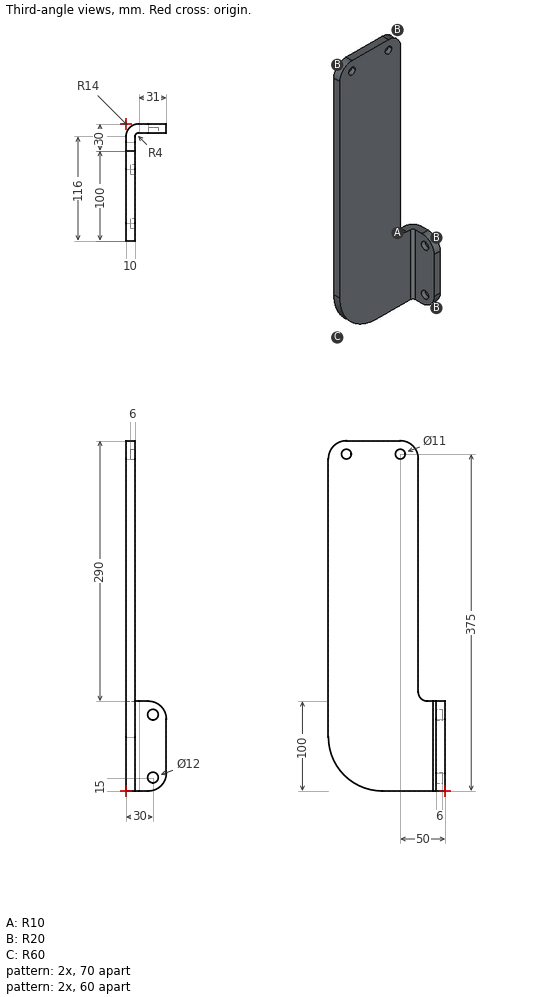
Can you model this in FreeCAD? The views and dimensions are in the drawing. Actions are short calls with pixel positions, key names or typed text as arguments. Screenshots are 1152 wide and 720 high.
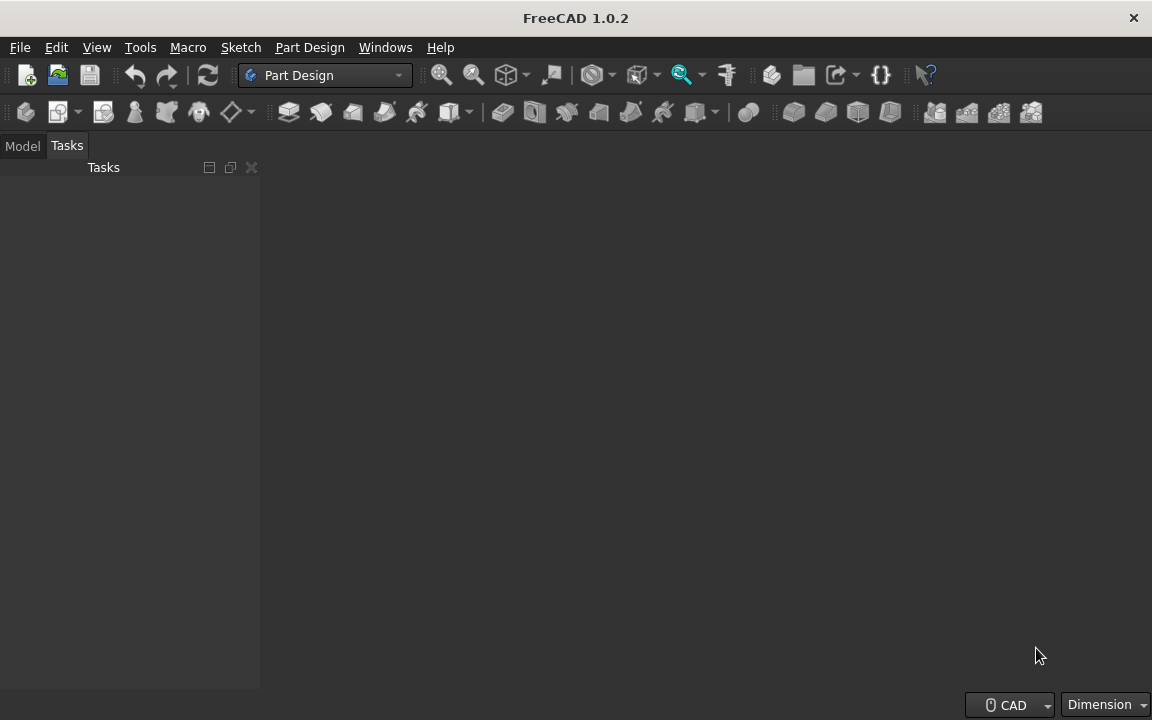
click(26, 76)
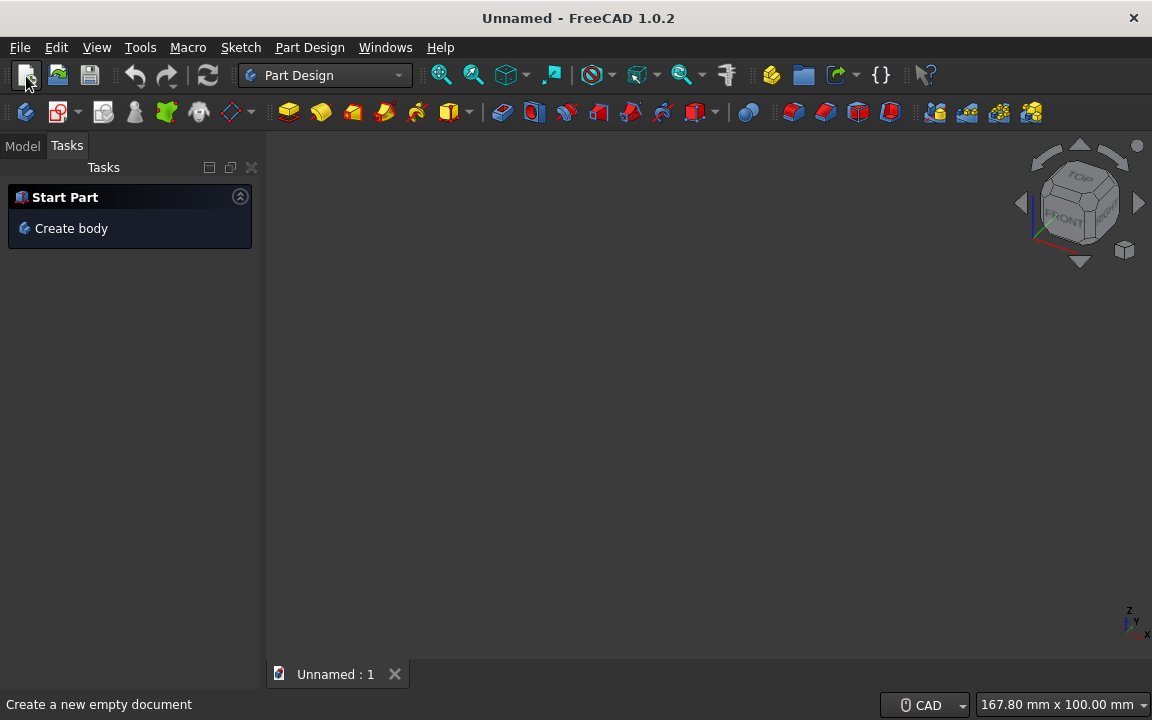
click(58, 112)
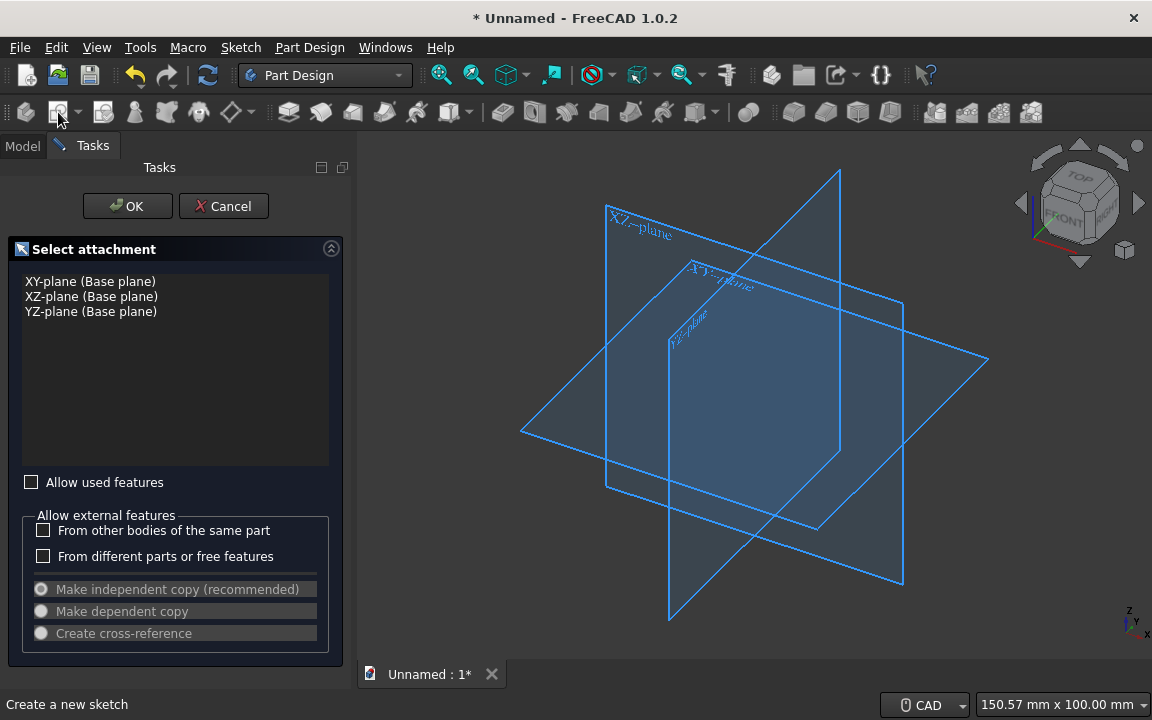
click(82, 282)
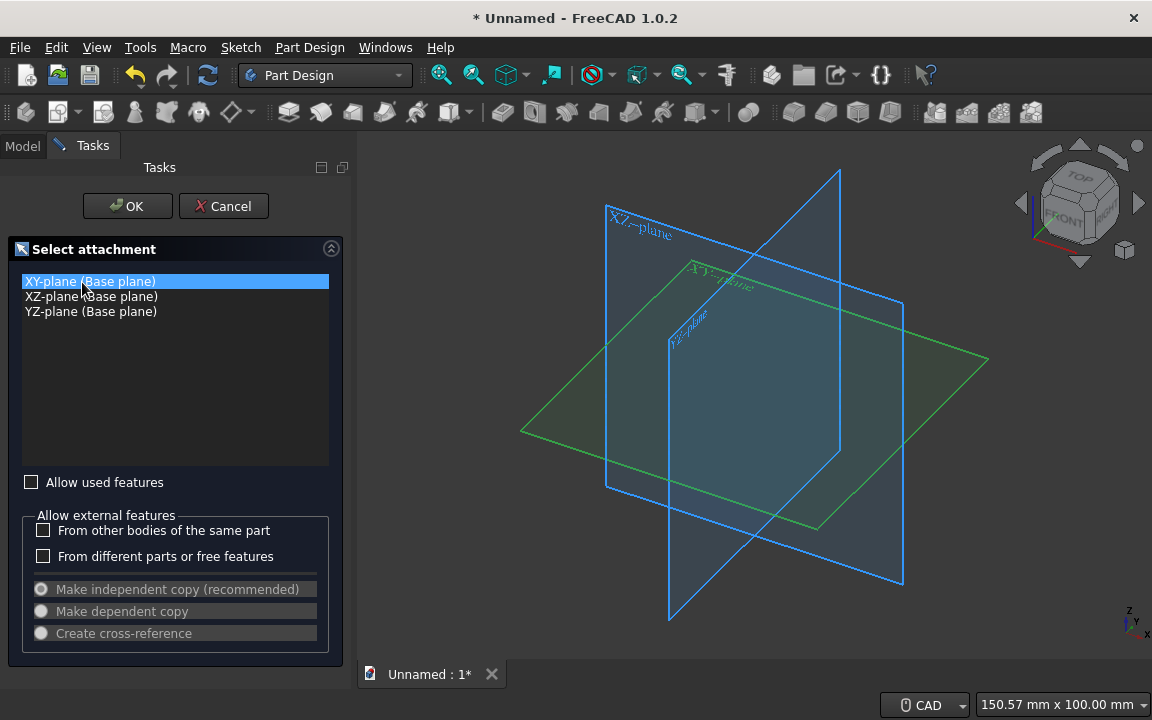
click(128, 206)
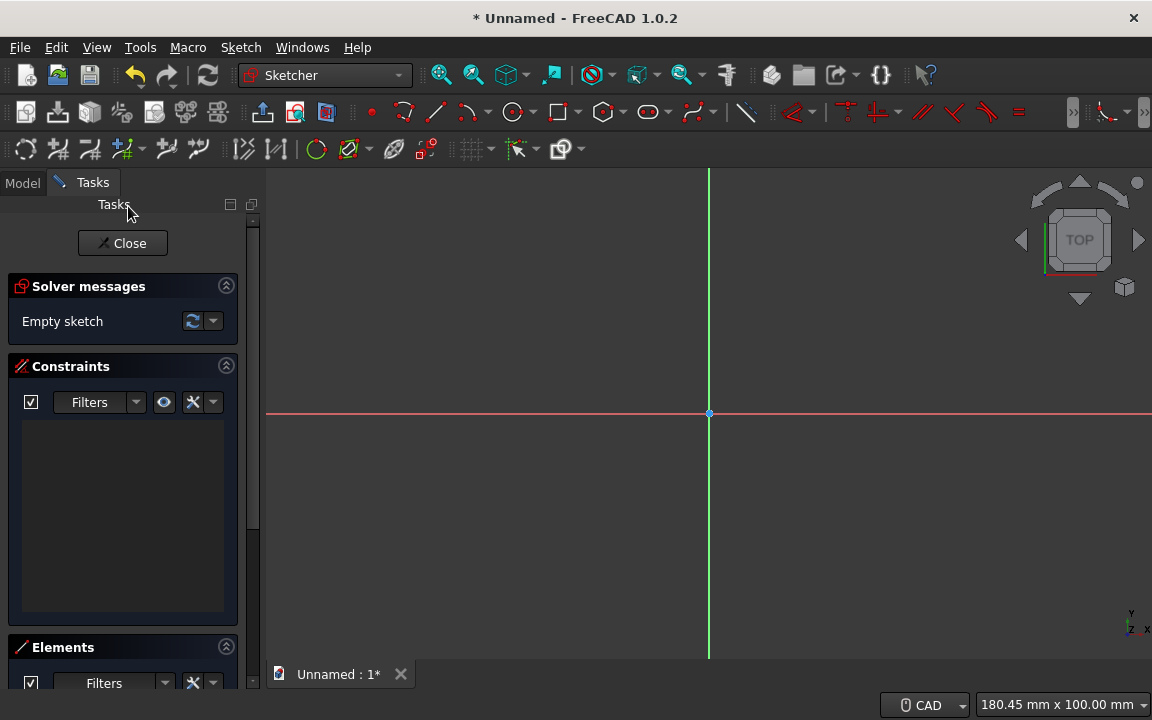
scroll(494, 196, down, 4)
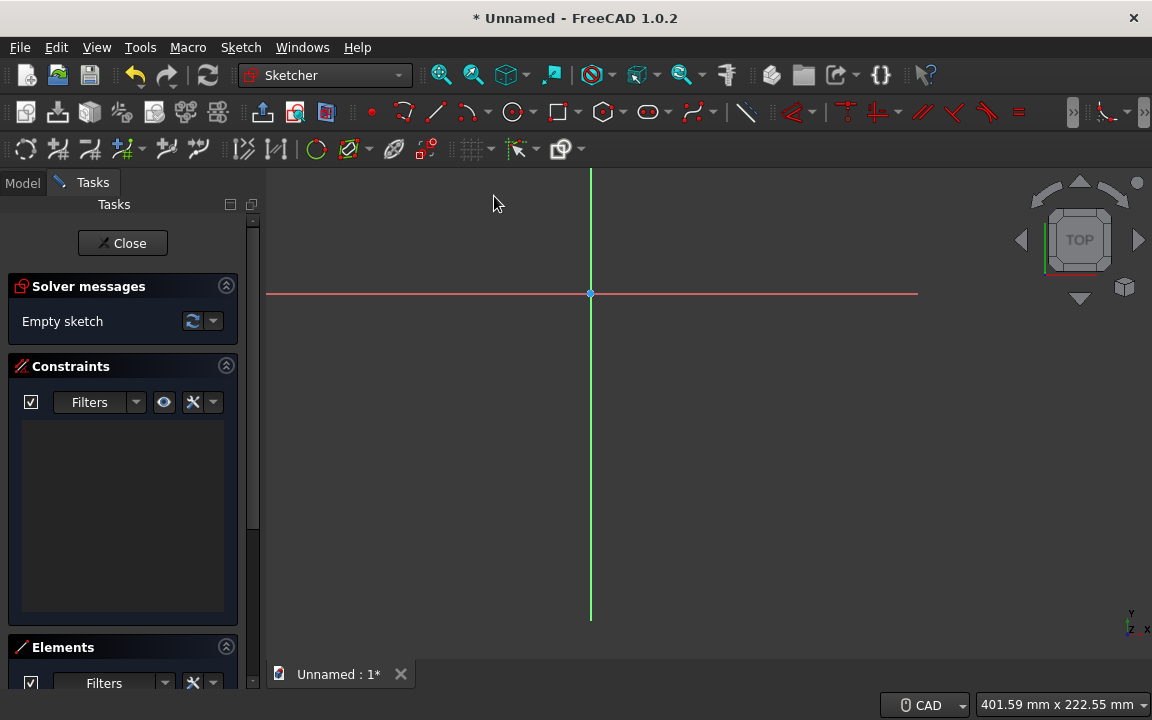
key(g)
key(m)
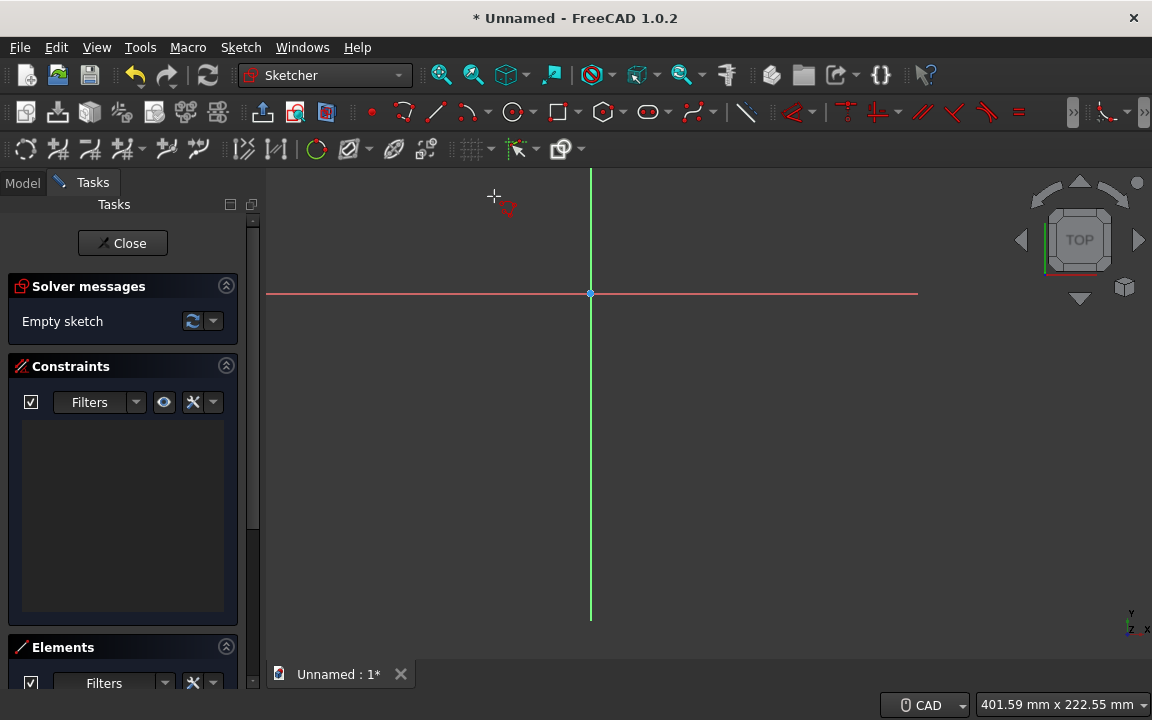
click(591, 325)
click(600, 581)
click(613, 581)
click(613, 325)
right_click(613, 325)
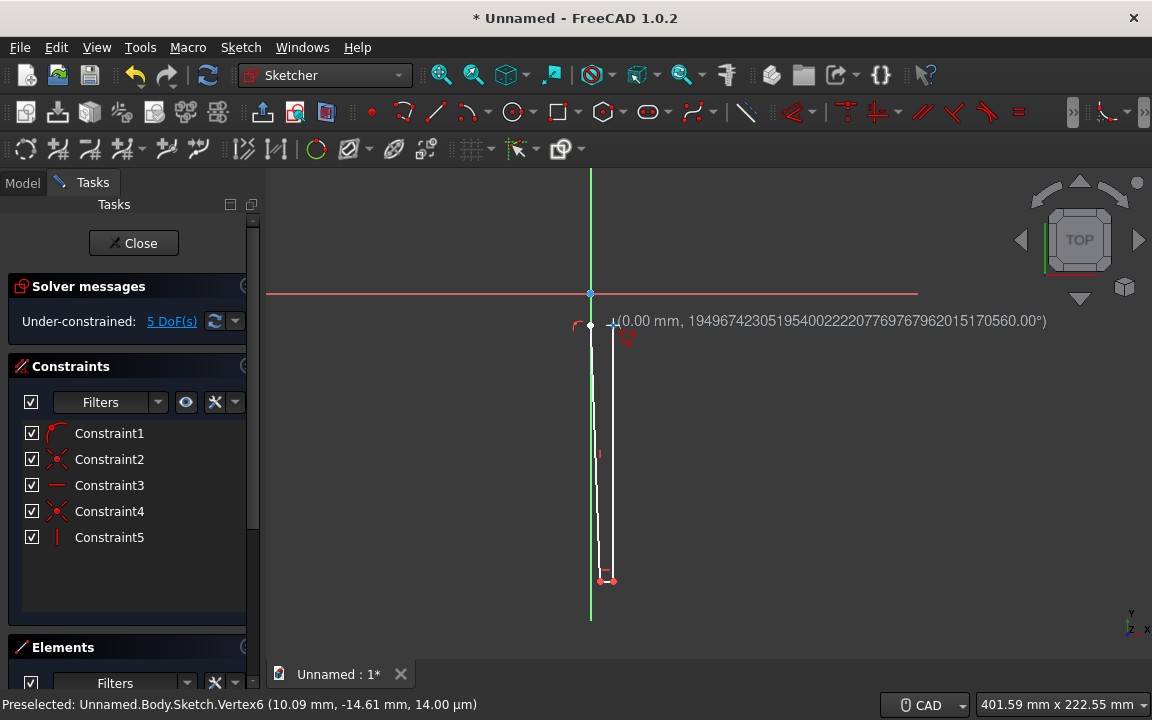
scroll(622, 316, up, 2)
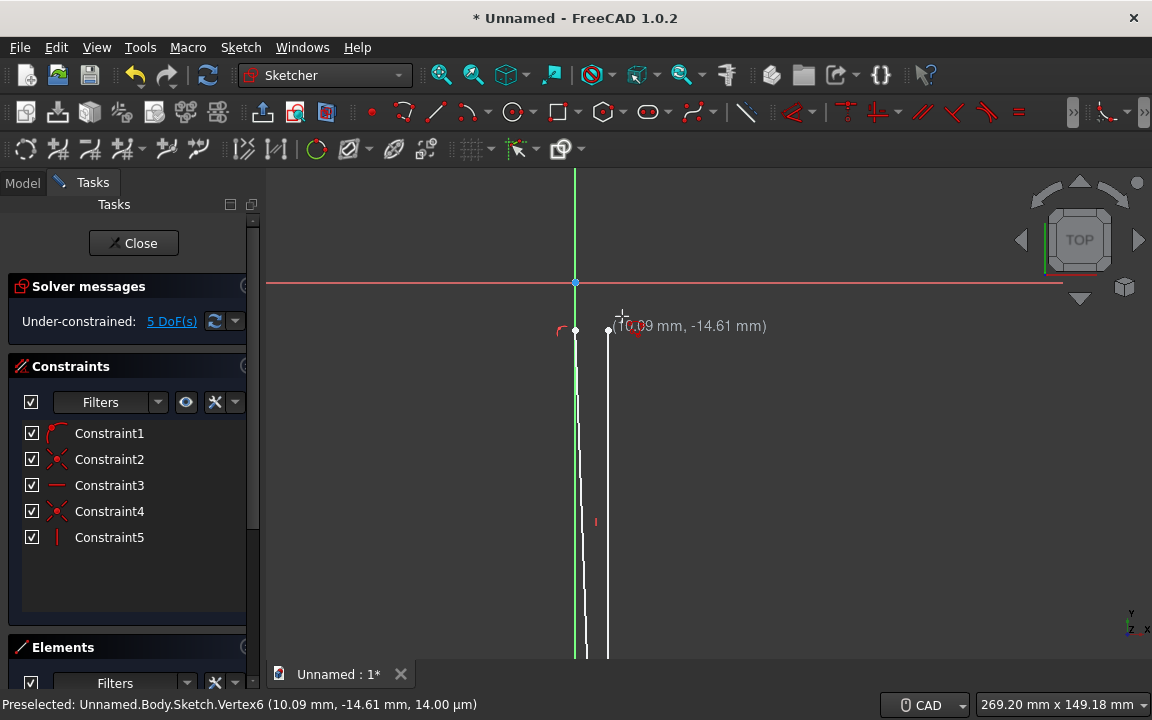
click(621, 316)
click(723, 316)
click(723, 283)
click(621, 292)
right_click(621, 292)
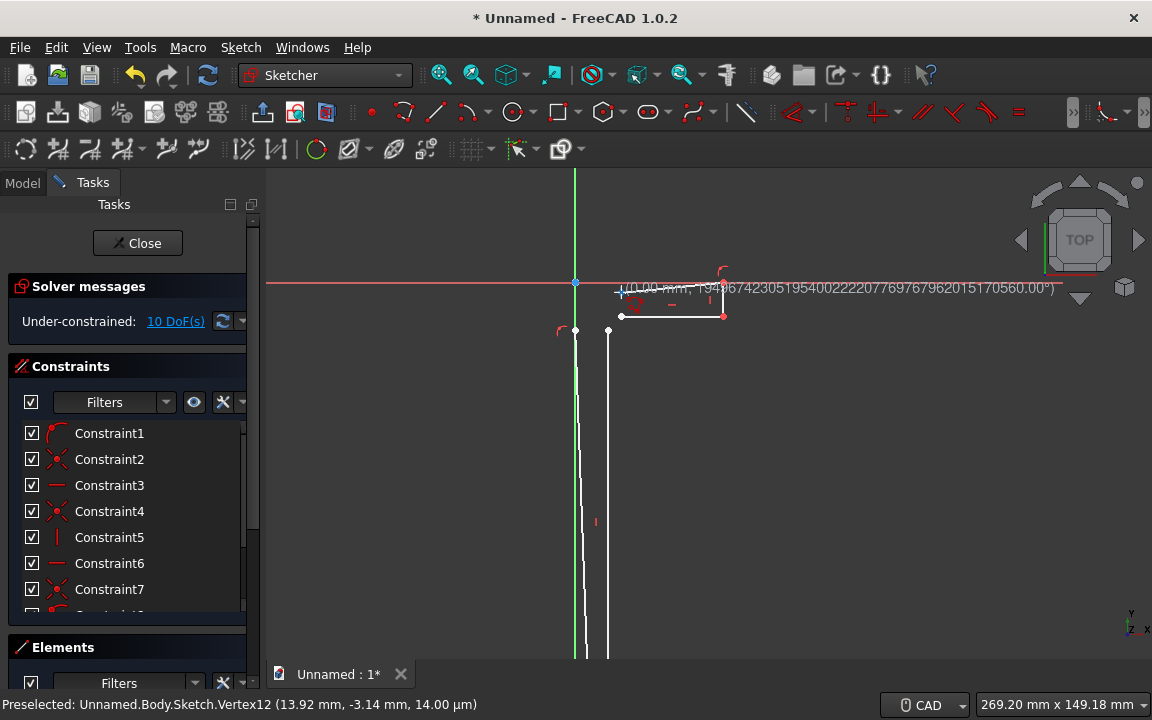
key(g)
key(3)
key(a)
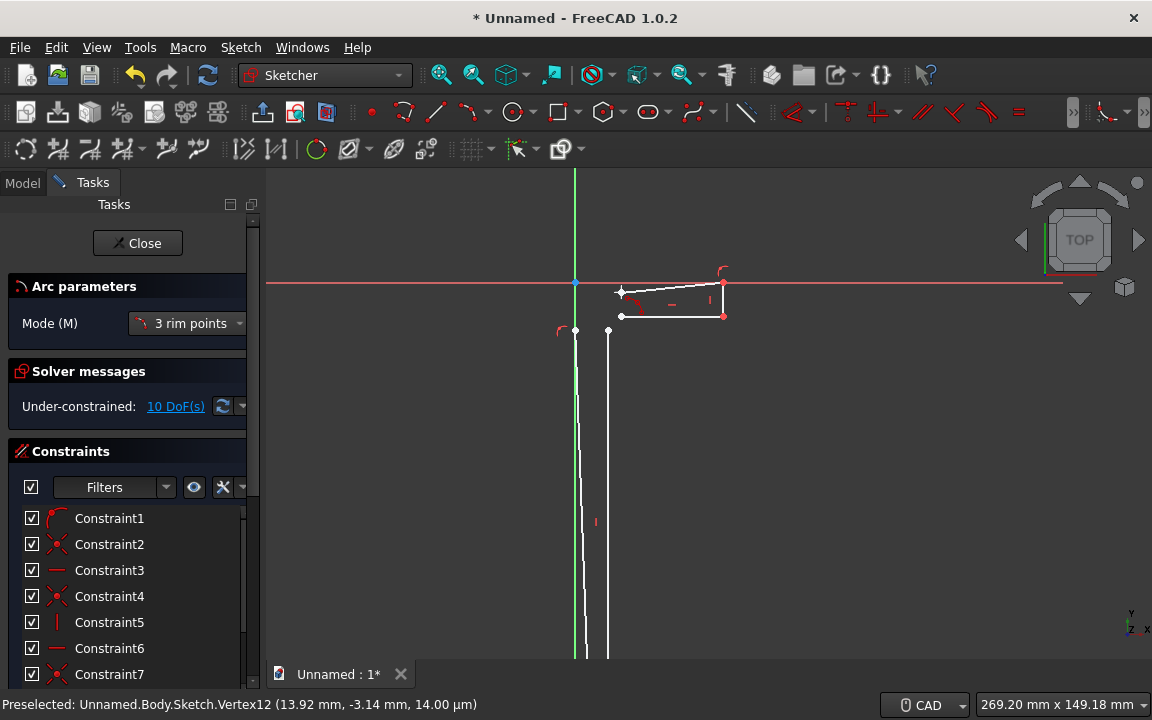
click(608, 331)
click(621, 317)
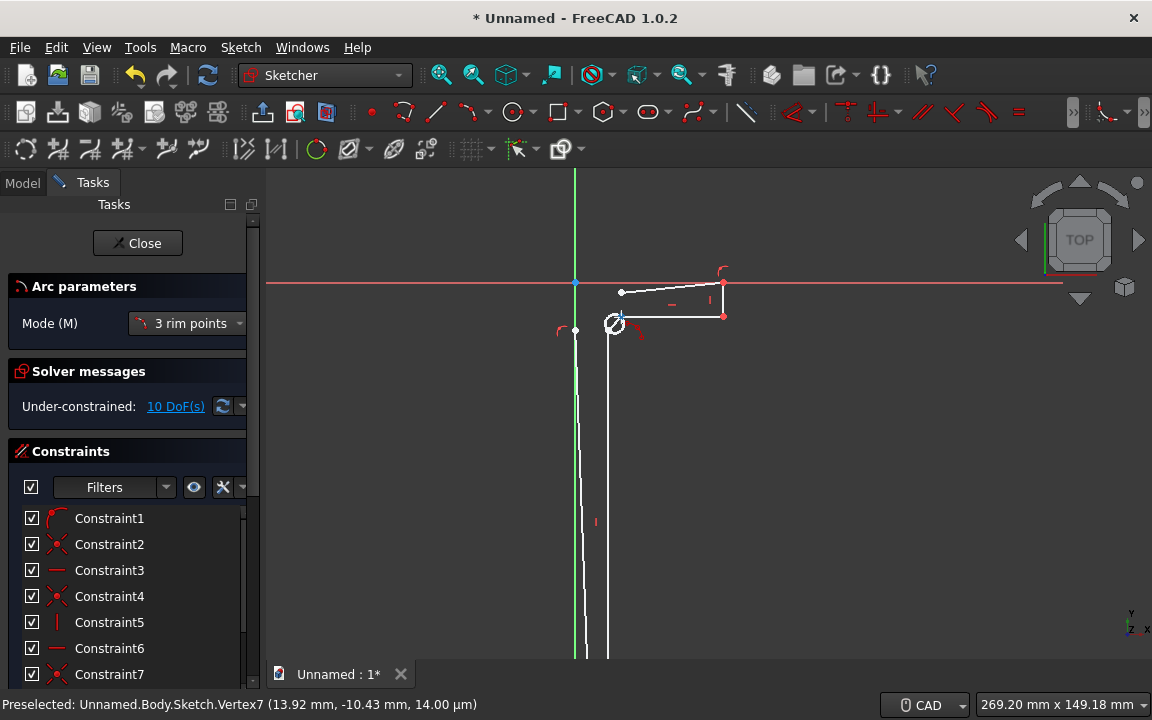
scroll(612, 319, up, 8)